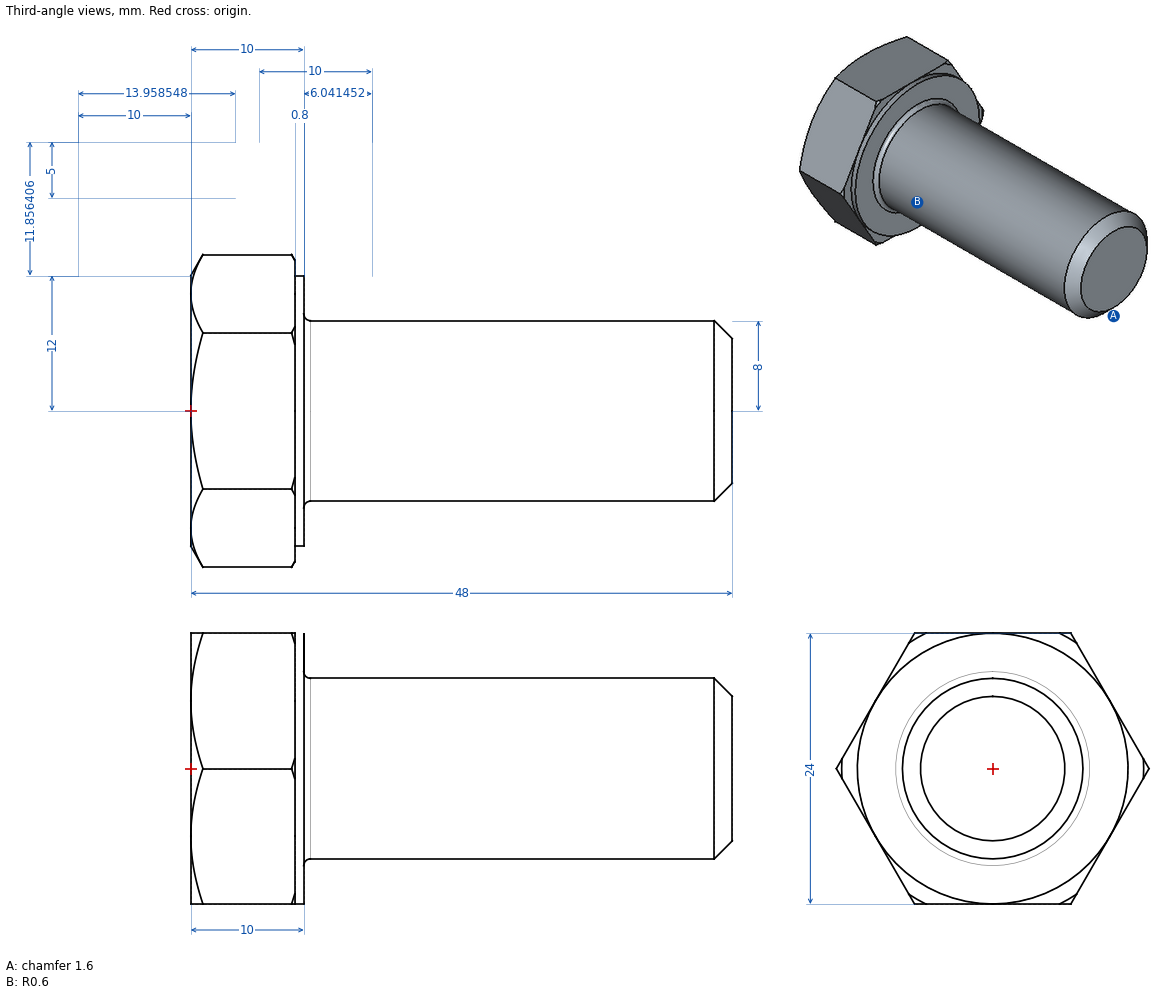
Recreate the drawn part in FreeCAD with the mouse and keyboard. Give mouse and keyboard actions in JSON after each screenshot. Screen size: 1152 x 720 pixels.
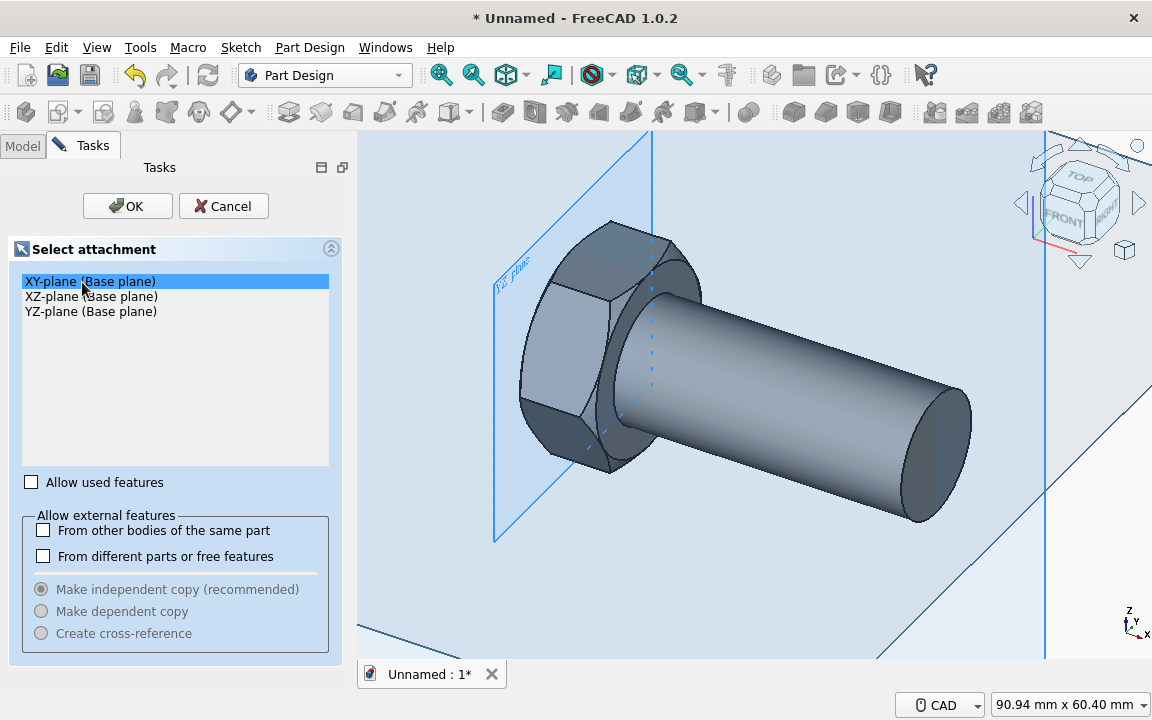
{"action": "left_click", "coordinate": [128, 206]}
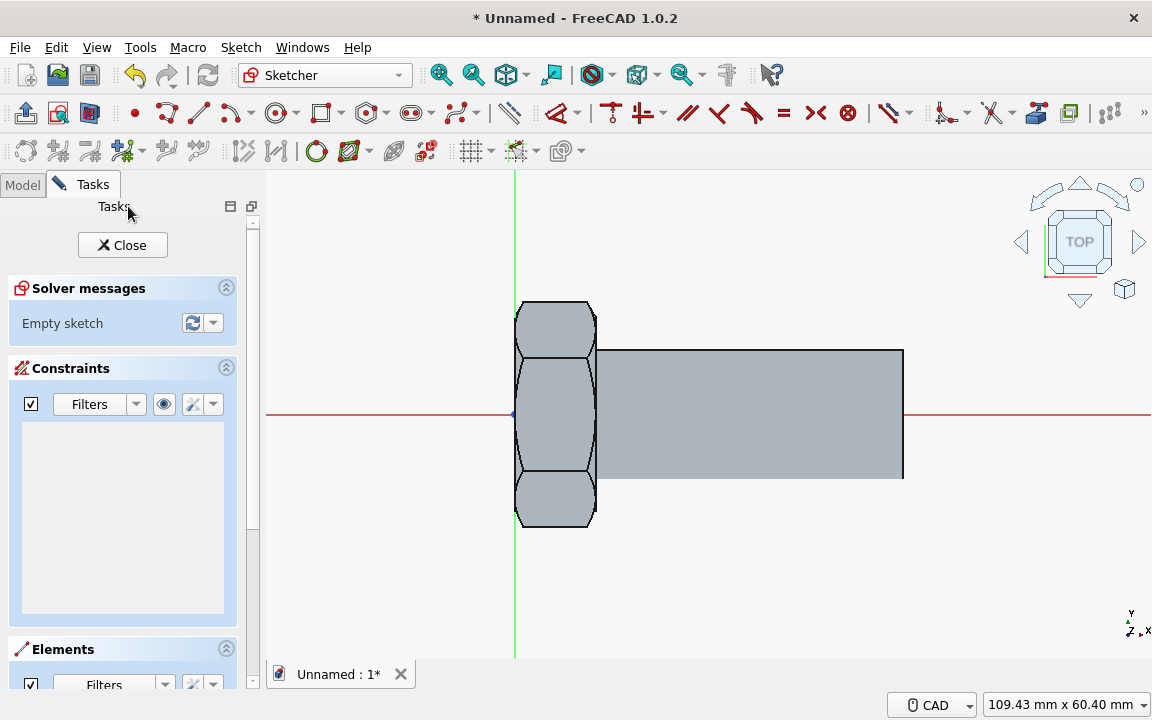
{"action": "left_click", "coordinate": [90, 114]}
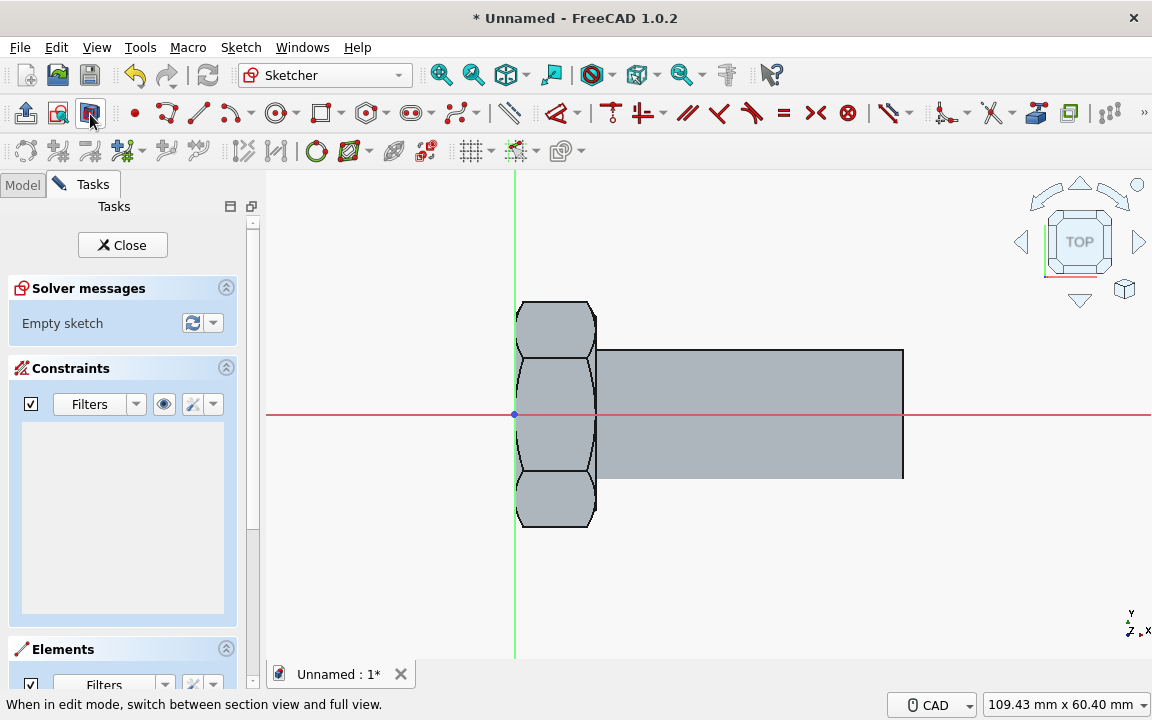
{"action": "scroll", "coordinate": [382, 198], "scroll_direction": "up", "scroll_amount": 2}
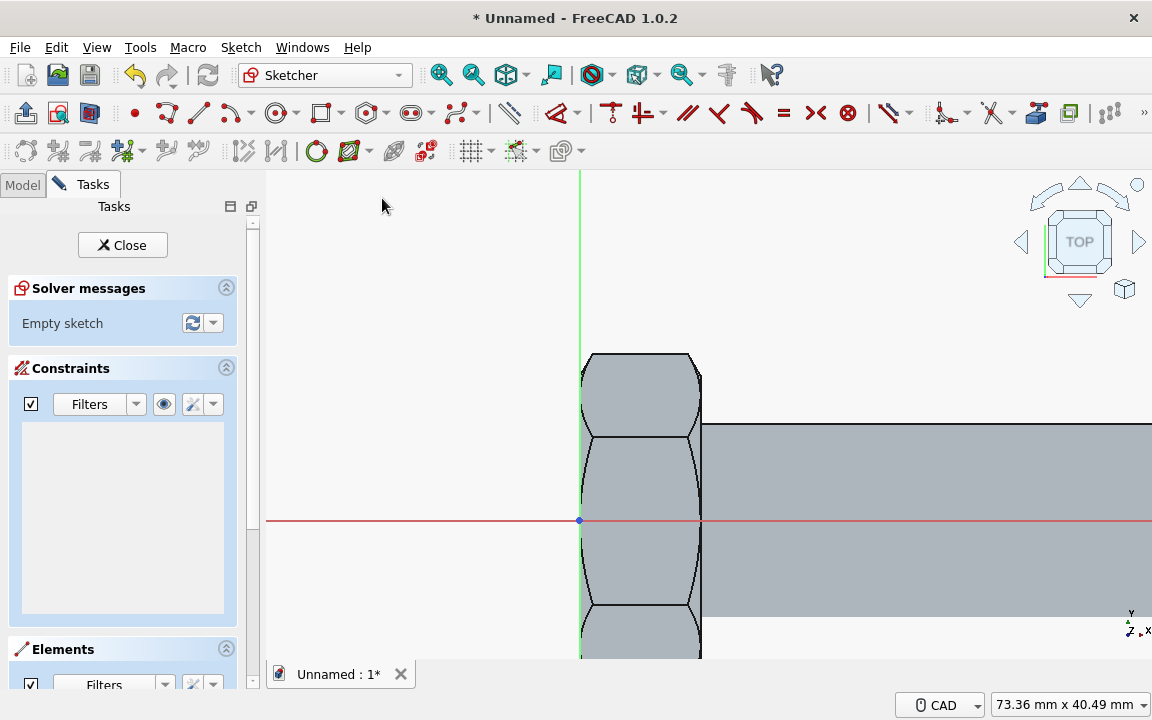
{"action": "left_click", "coordinate": [322, 114]}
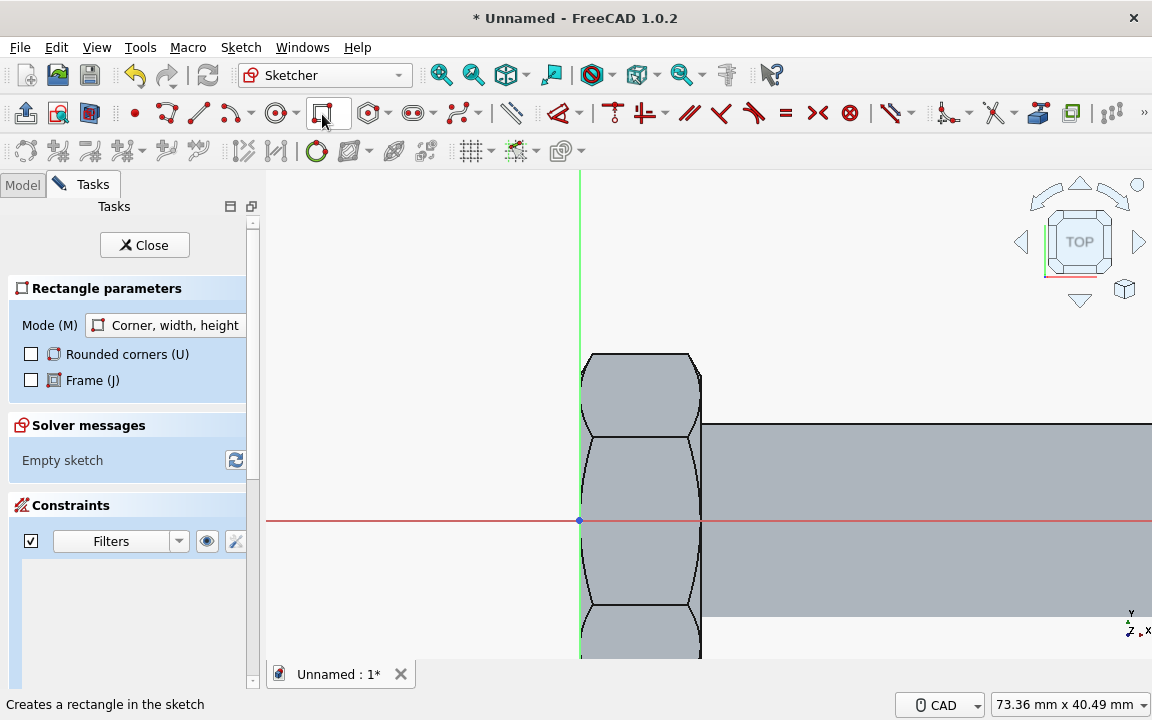
{"action": "scroll", "coordinate": [691, 233], "scroll_direction": "up", "scroll_amount": 3}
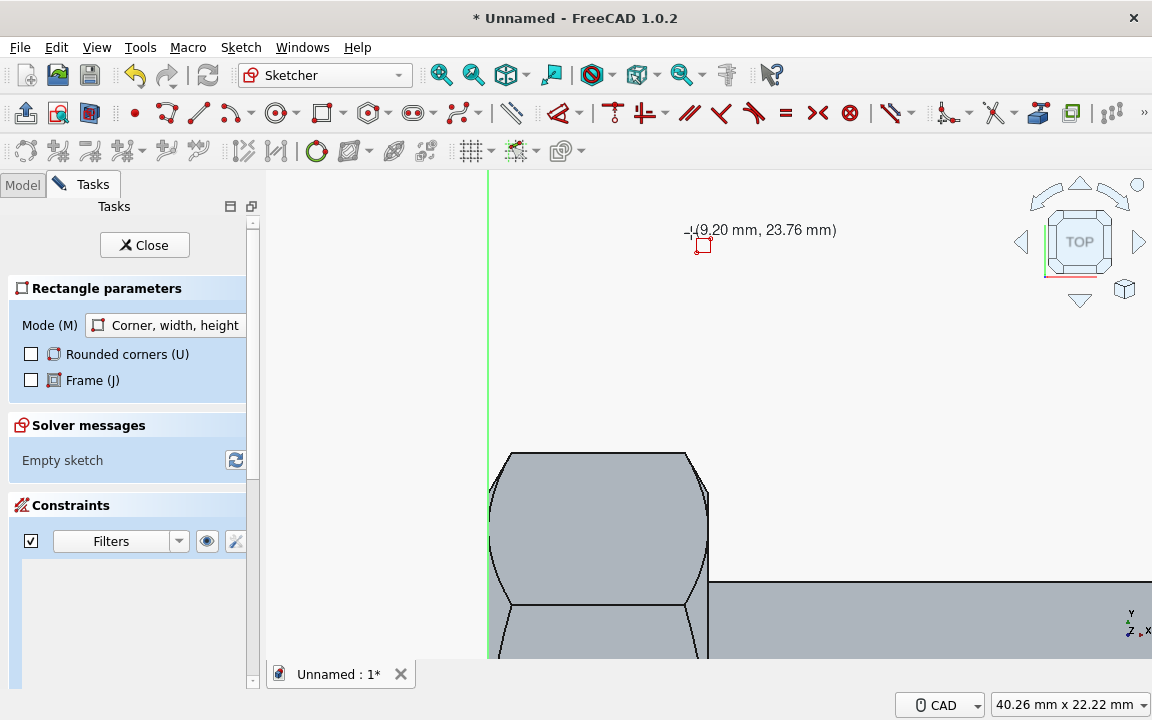
{"action": "left_click", "coordinate": [691, 233]}
{"action": "mouse_move", "coordinate": [708, 493]}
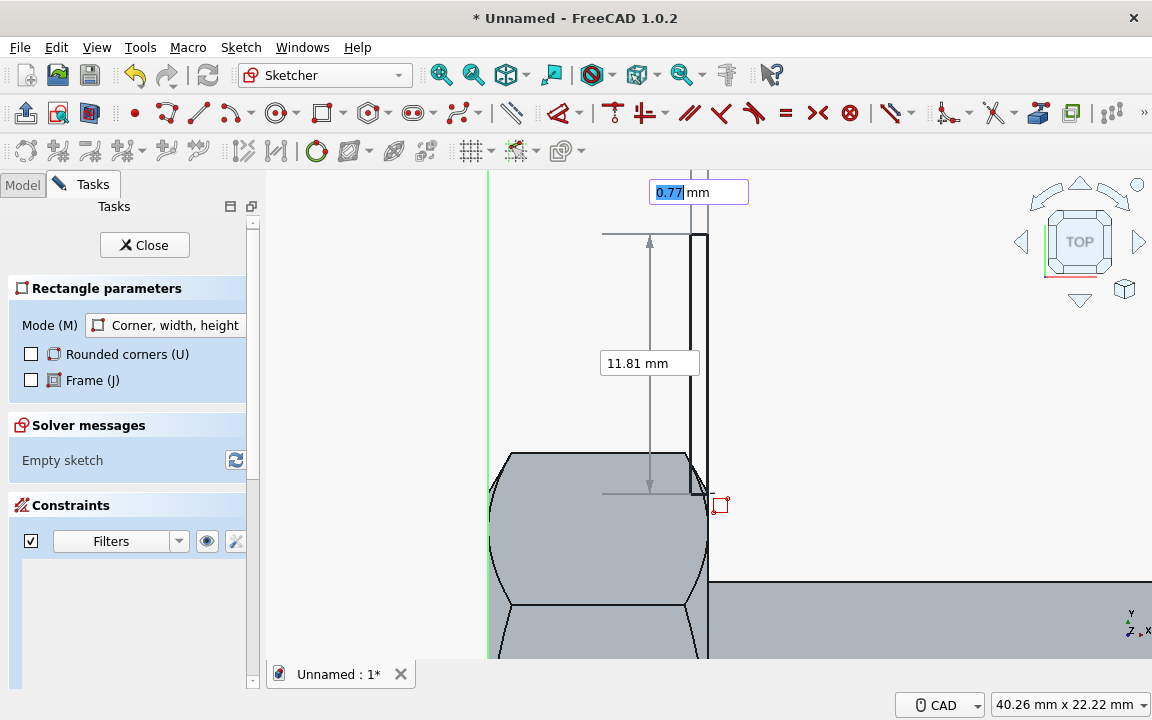
{"action": "type", "text": "0.8"}
{"action": "key", "text": "Tab"}
{"action": "type", "text": "11.856406"}
{"action": "key", "text": "Return"}
{"action": "key", "text": "Escape"}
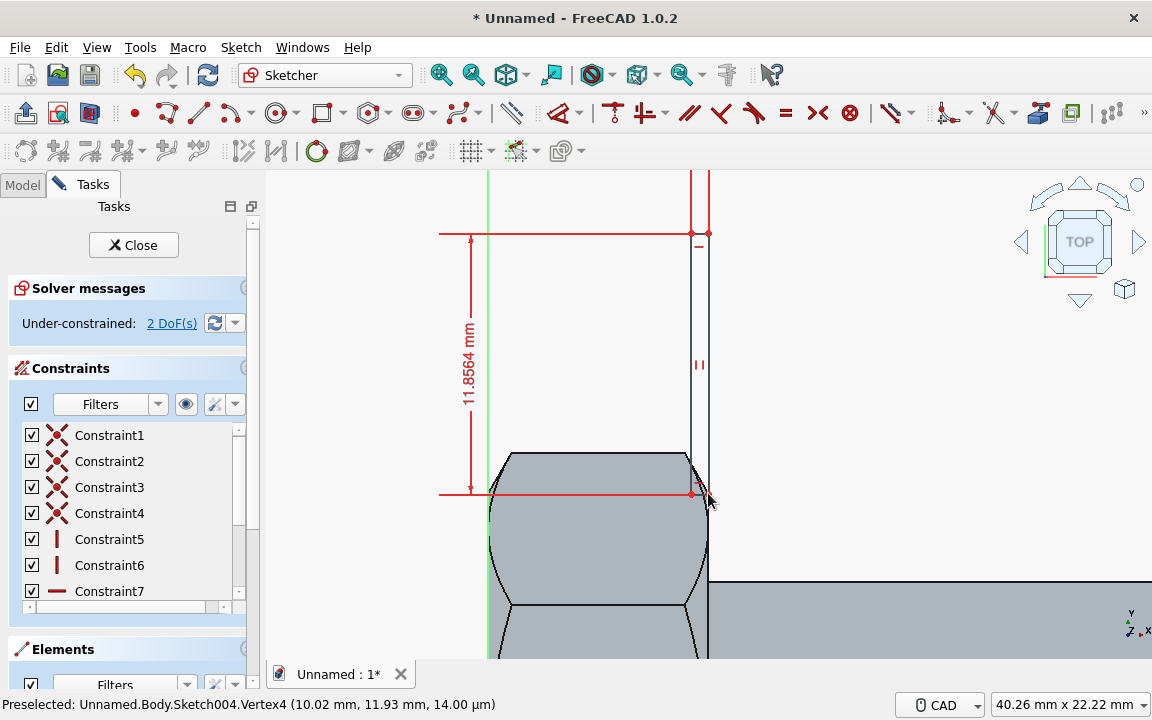
{"action": "left_click", "coordinate": [558, 114]}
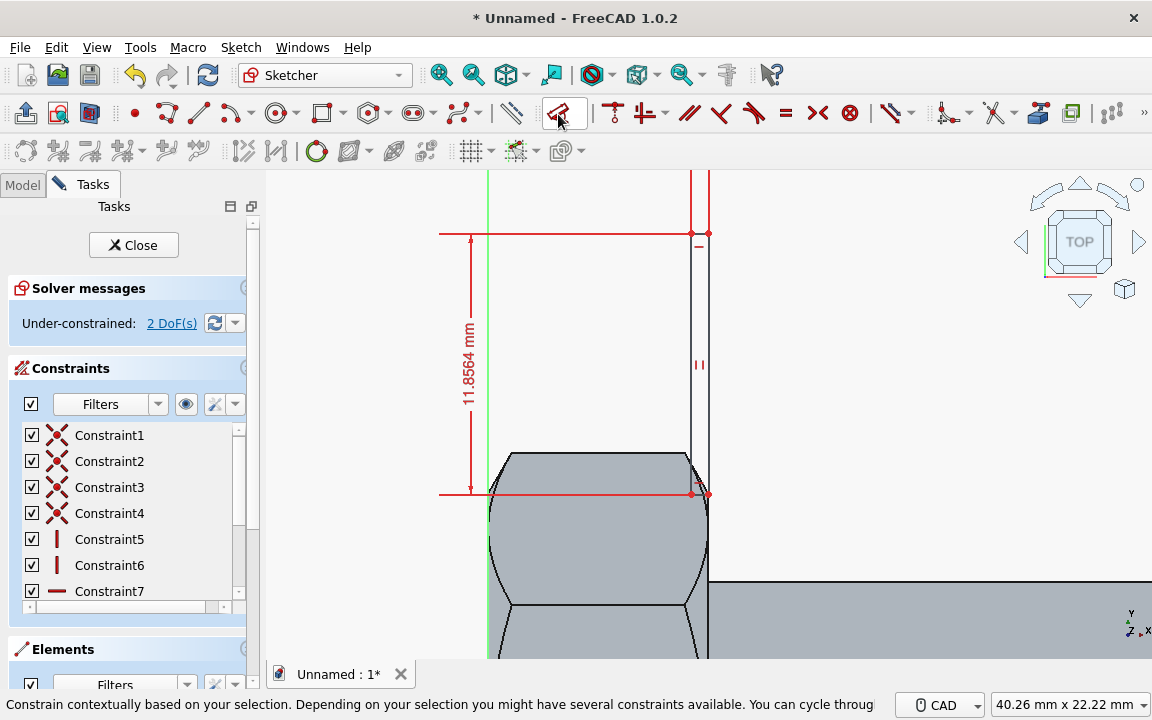
{"action": "left_click", "coordinate": [691, 495]}
{"action": "left_click", "coordinate": [454, 563]}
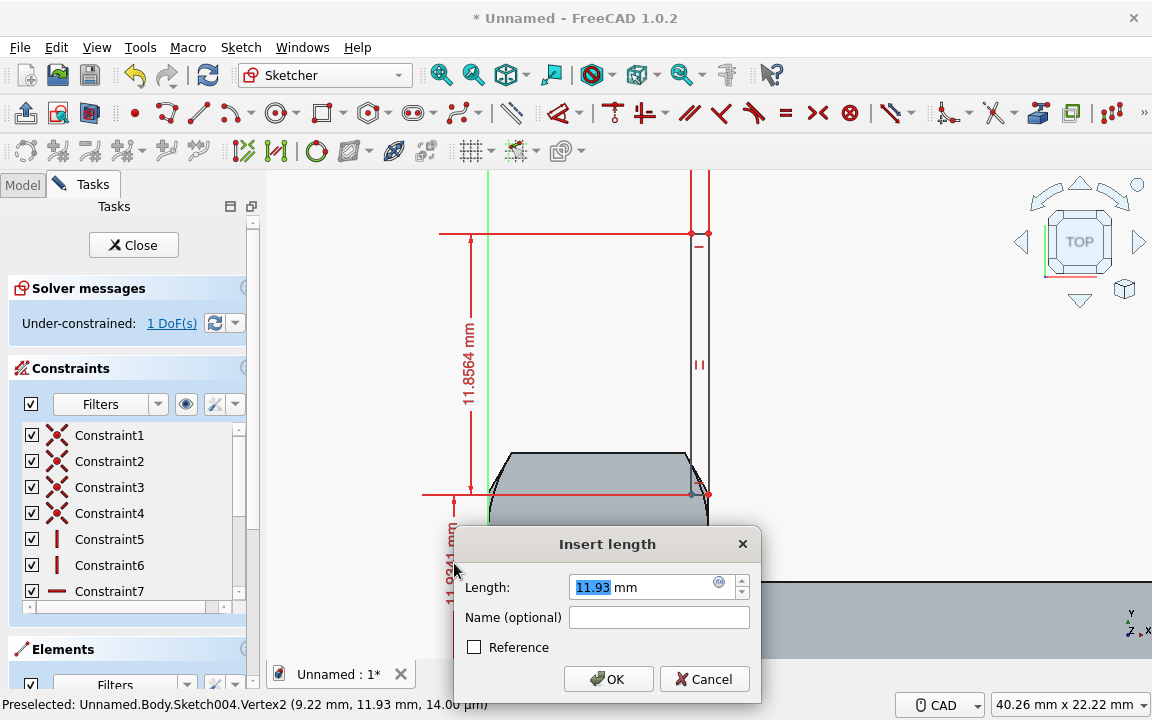
{"action": "type", "text": "12"}
{"action": "key", "text": "Return"}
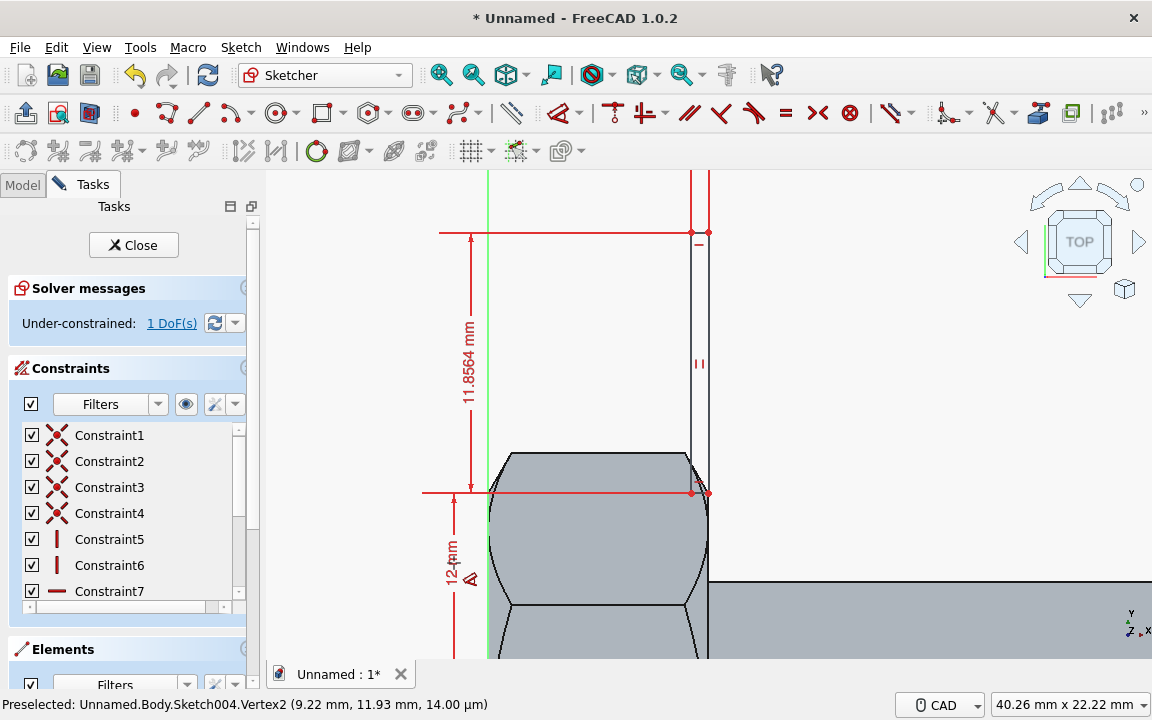
{"action": "left_click", "coordinate": [709, 493]}
{"action": "left_click", "coordinate": [598, 459]}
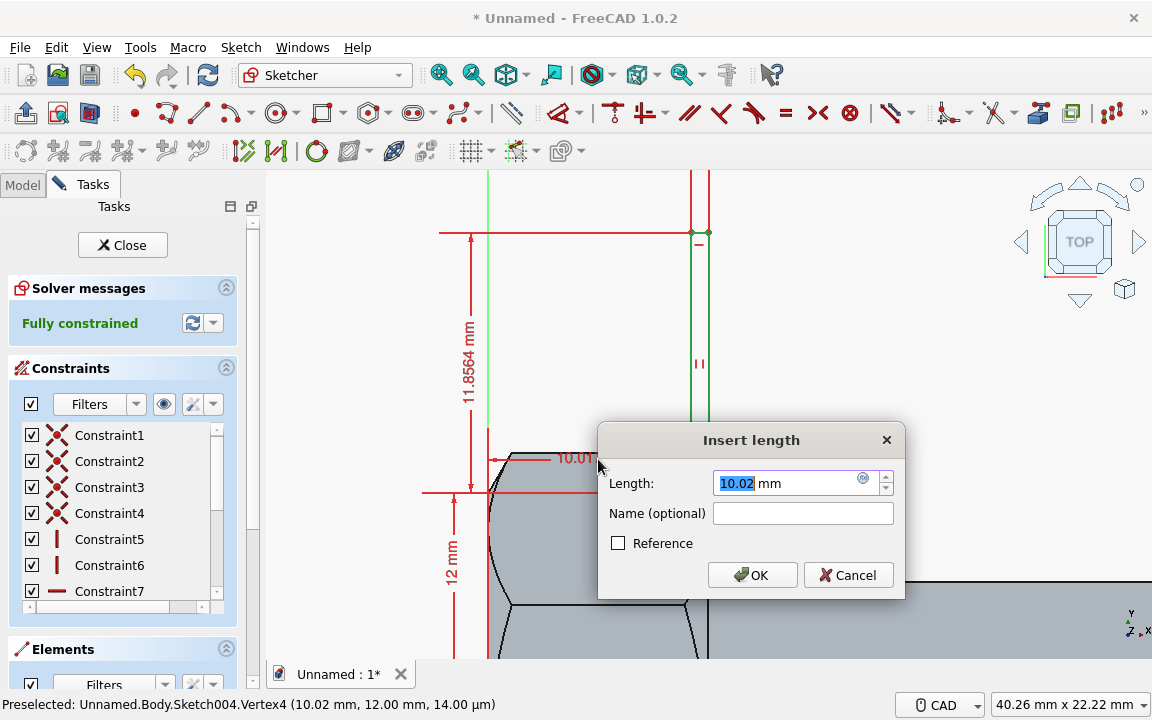
{"action": "type", "text": "10"}
{"action": "key", "text": "Return"}
{"action": "key", "text": "Escape"}